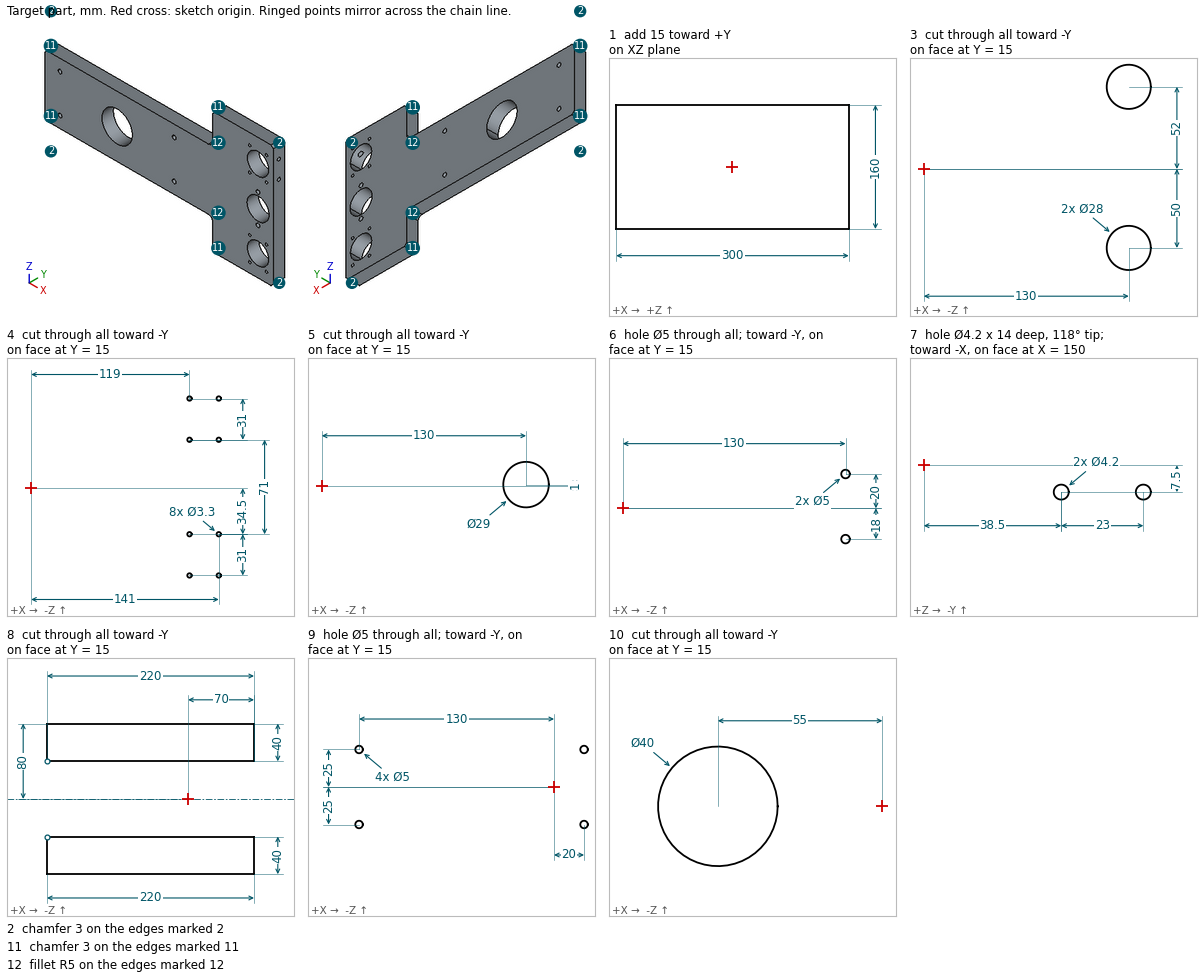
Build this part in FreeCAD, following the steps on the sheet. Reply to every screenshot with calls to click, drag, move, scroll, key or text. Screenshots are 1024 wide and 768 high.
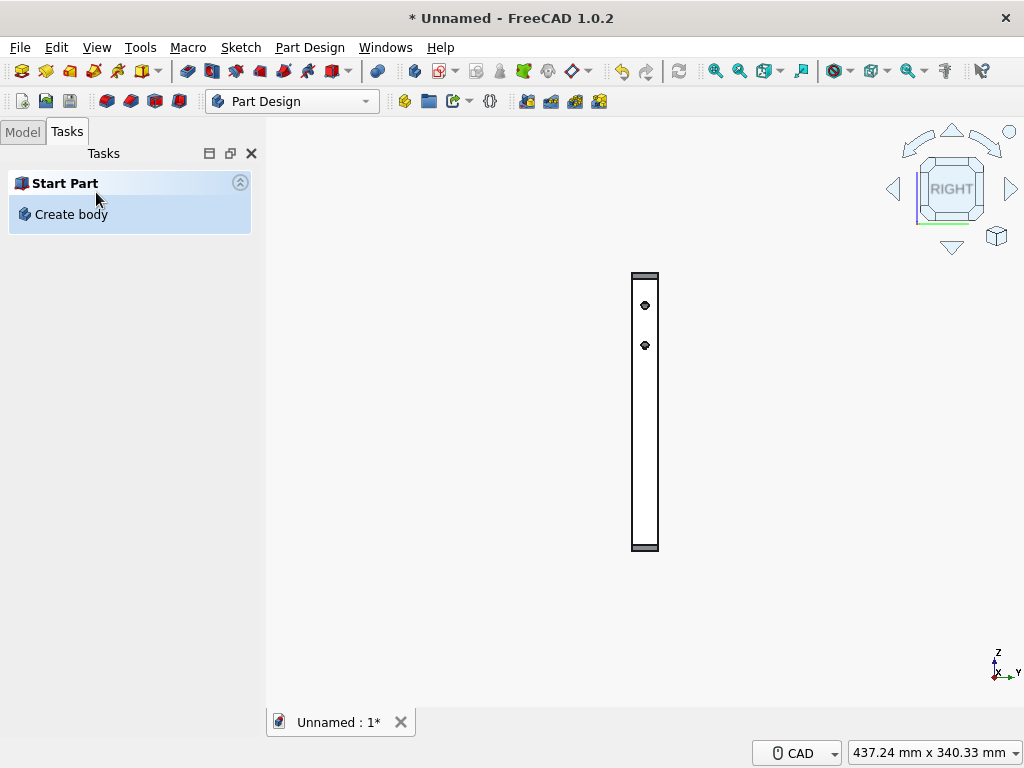
key(5)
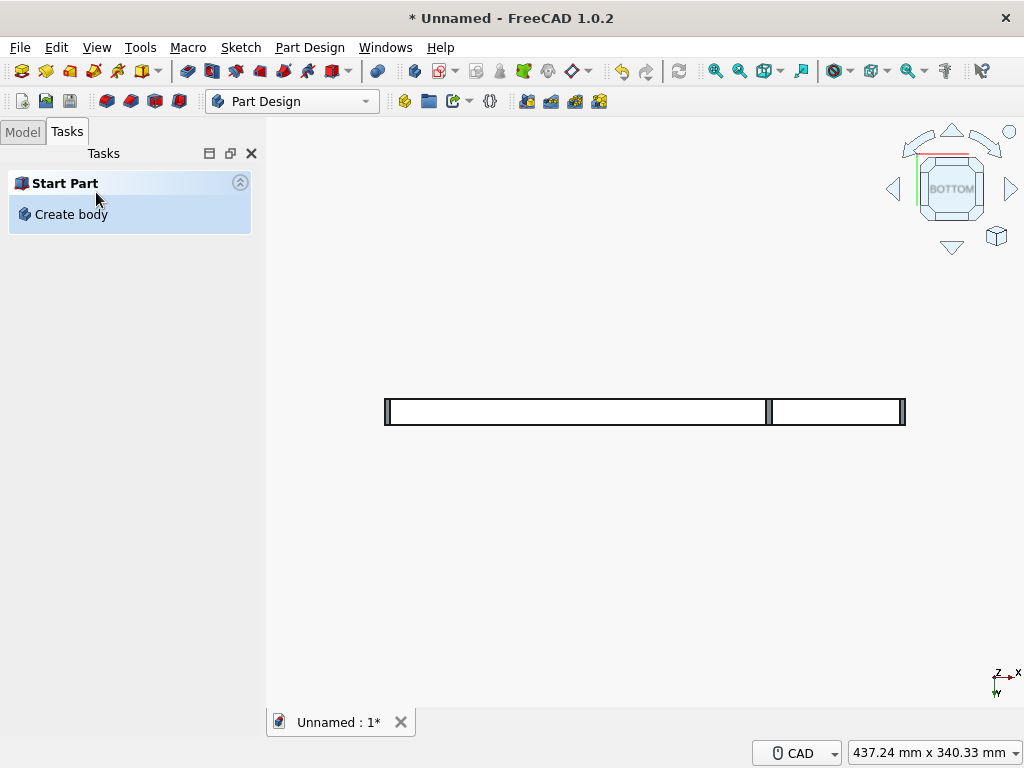
key(4)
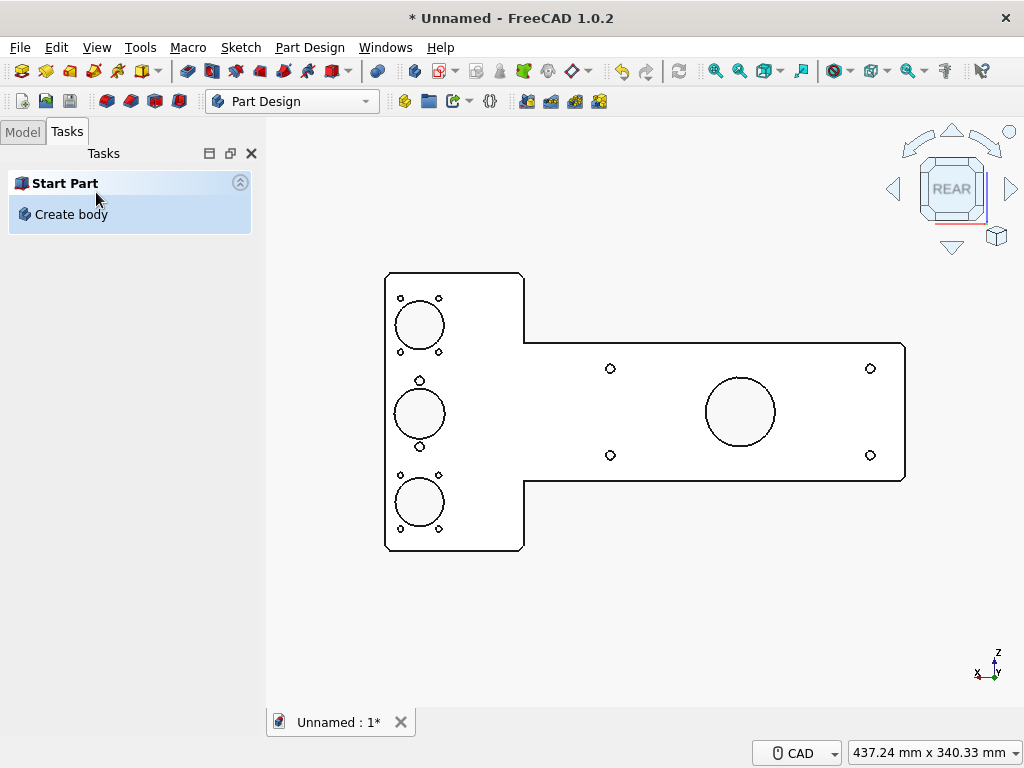
key(6)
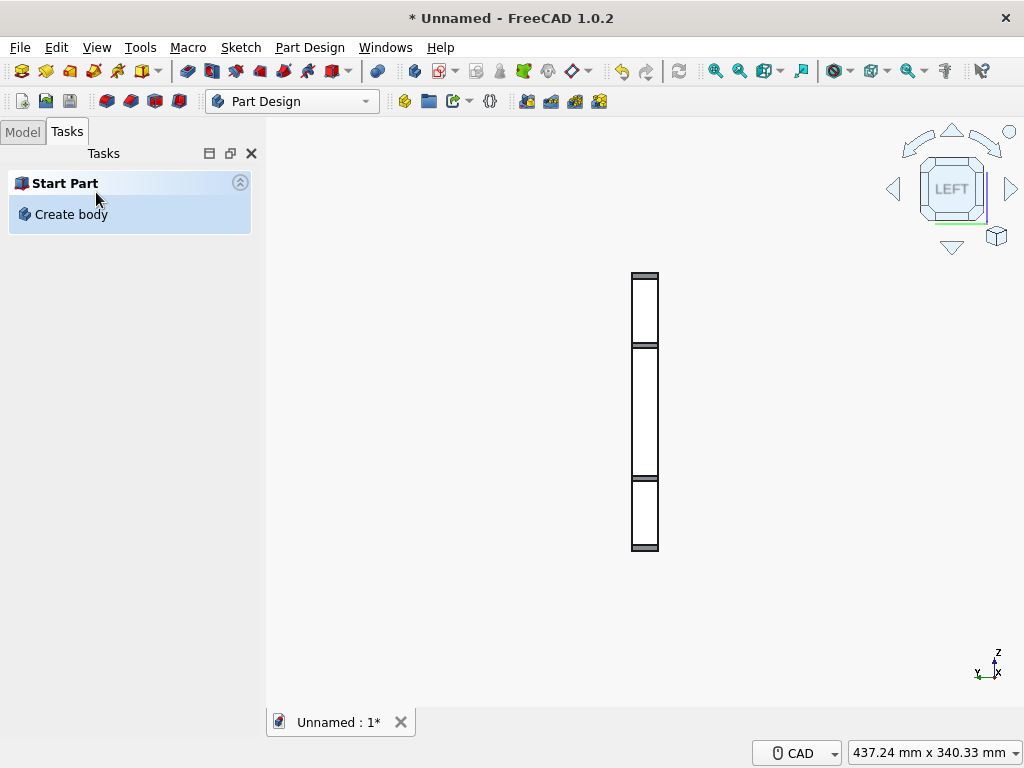
key(v)
key(3)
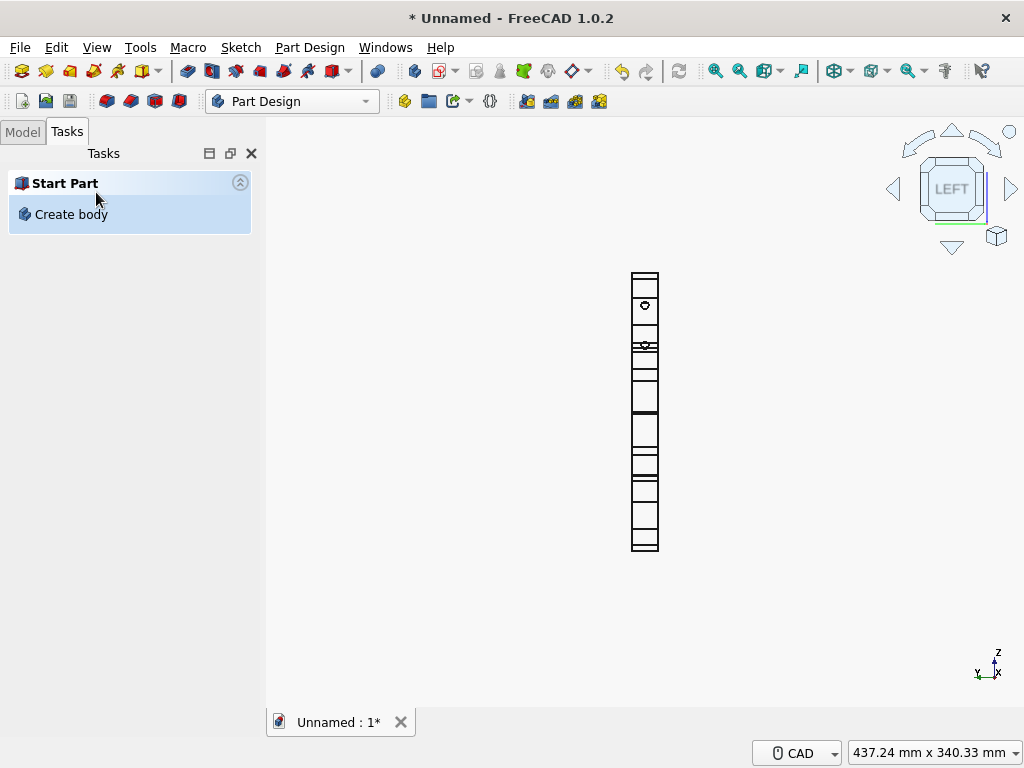
key(0)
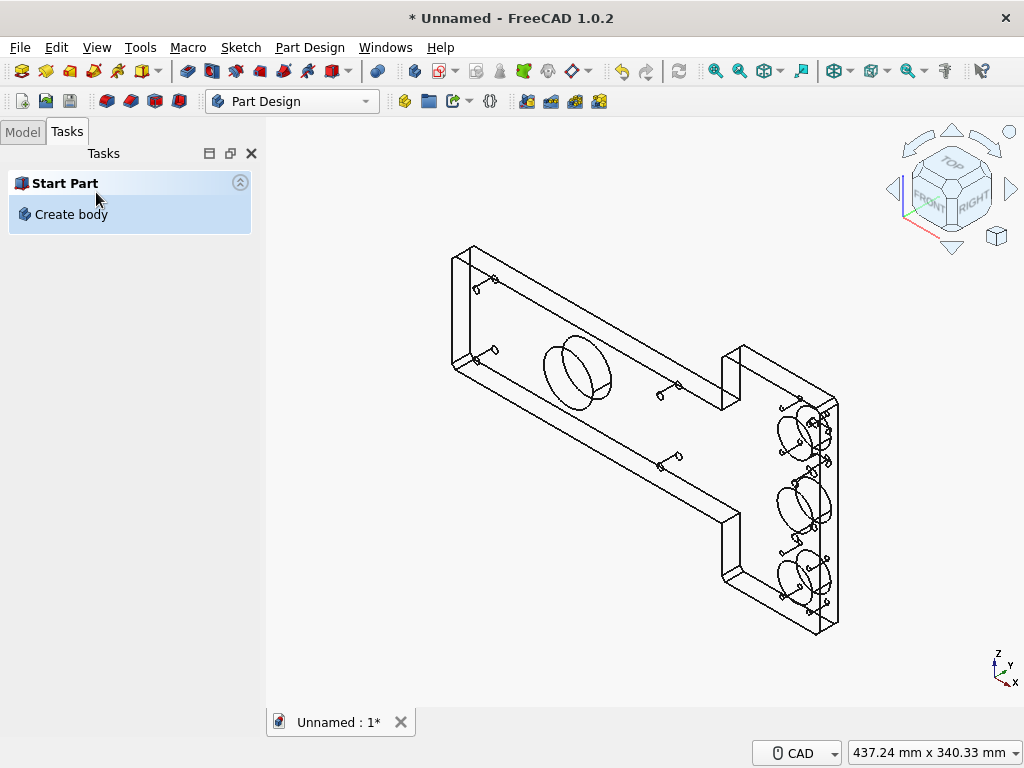
click(731, 517)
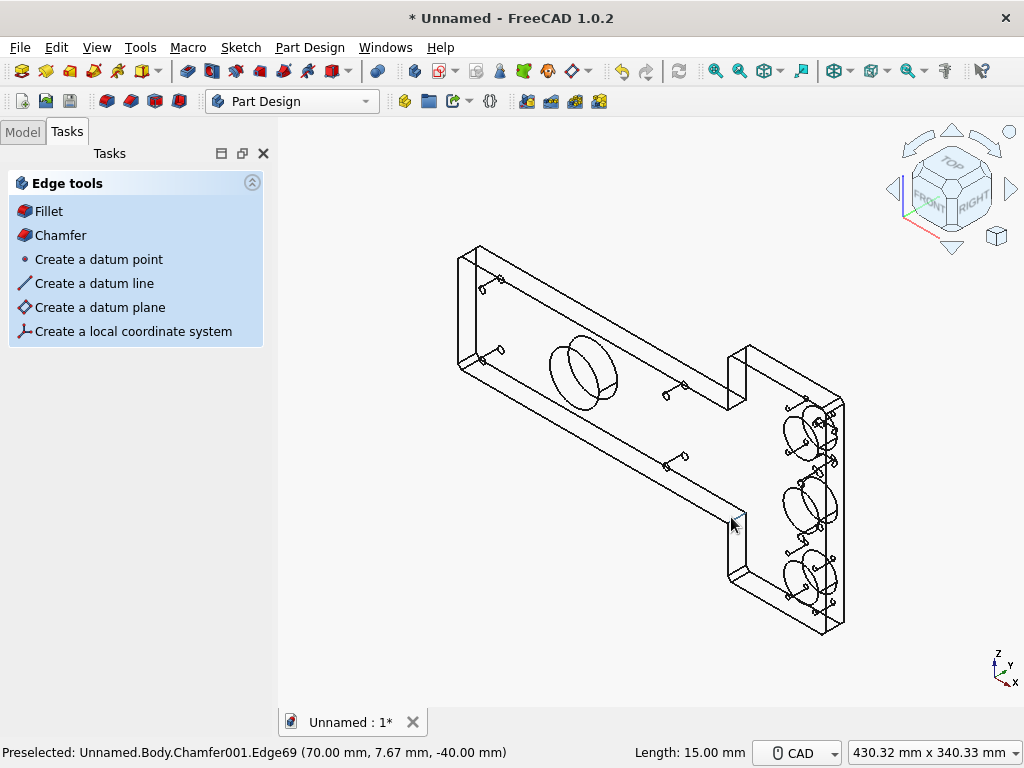
click(737, 404, ctrl)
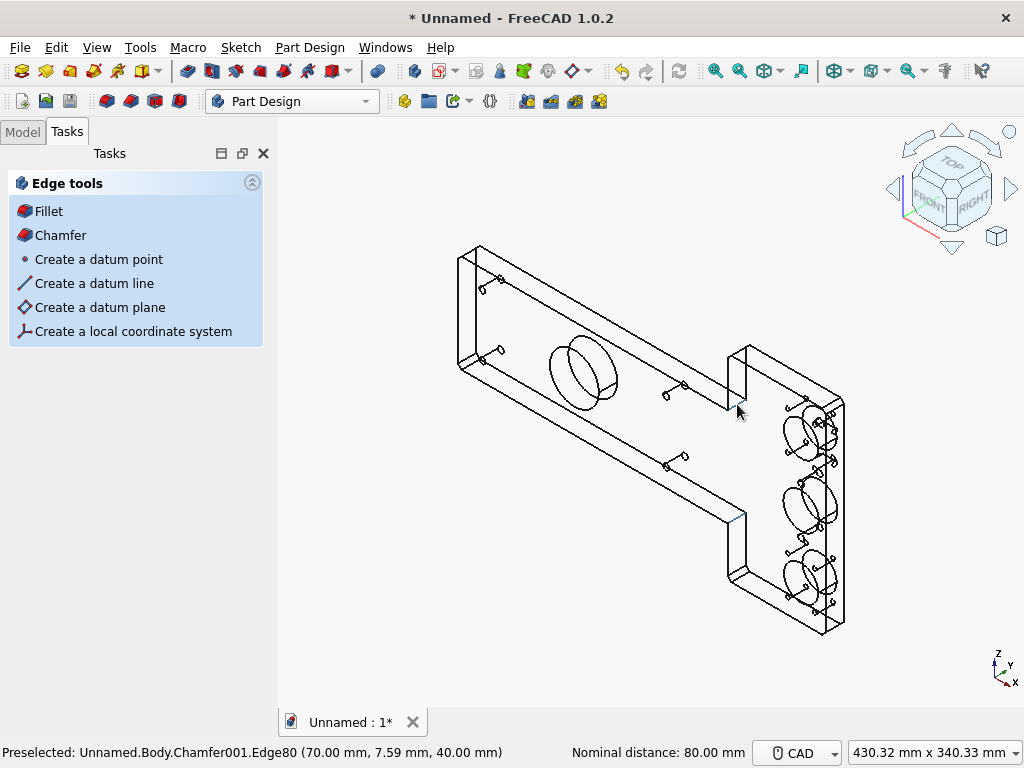
key(v)
key(1)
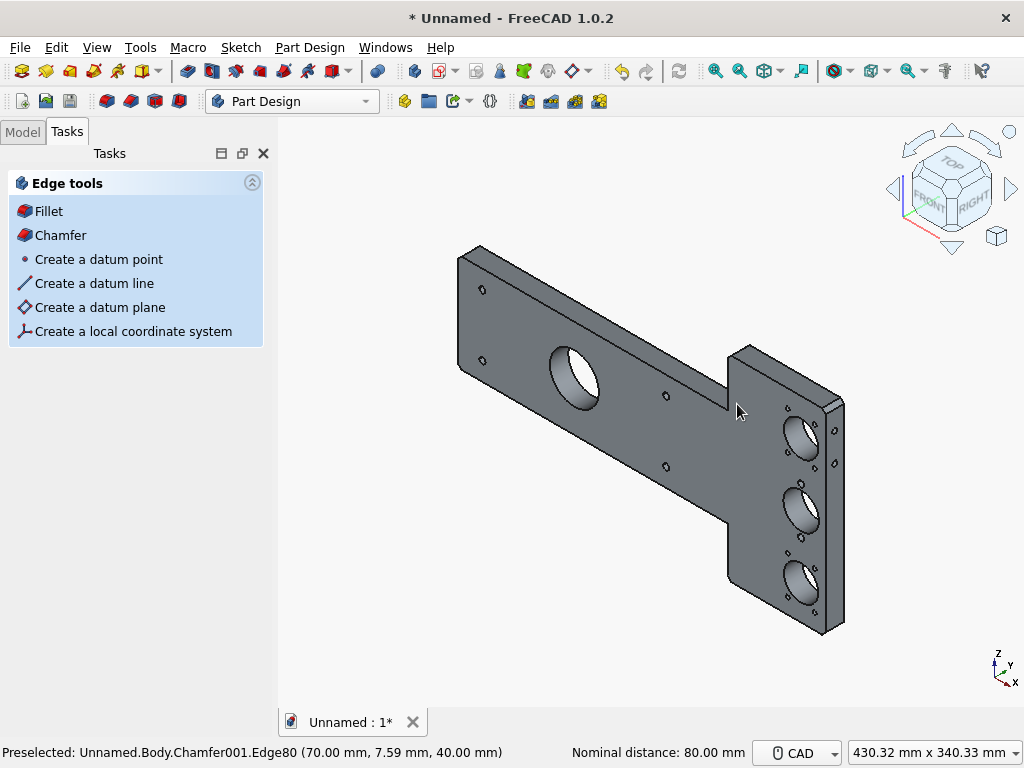
click(108, 102)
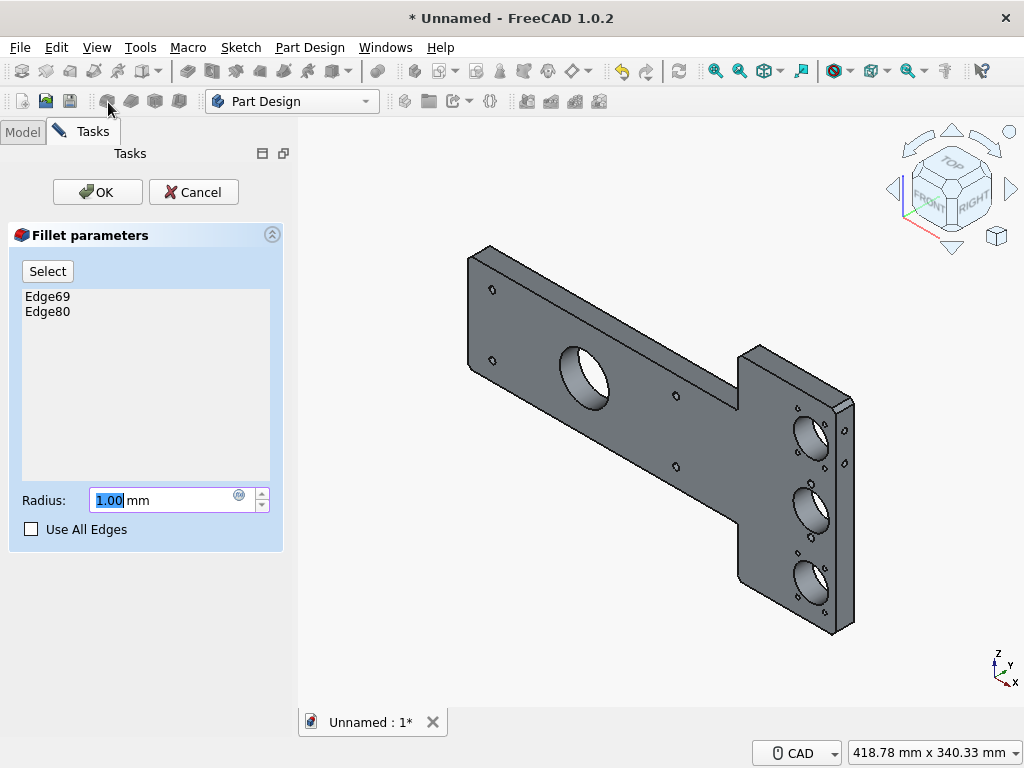
text(5)
key(Tab)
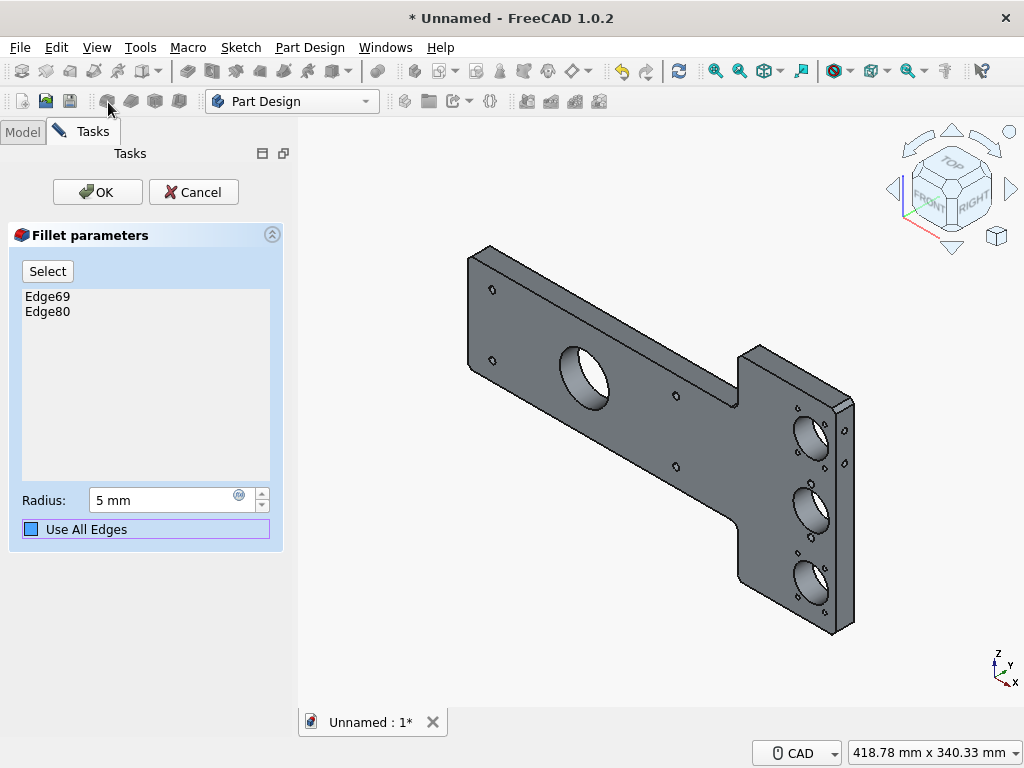
click(98, 192)